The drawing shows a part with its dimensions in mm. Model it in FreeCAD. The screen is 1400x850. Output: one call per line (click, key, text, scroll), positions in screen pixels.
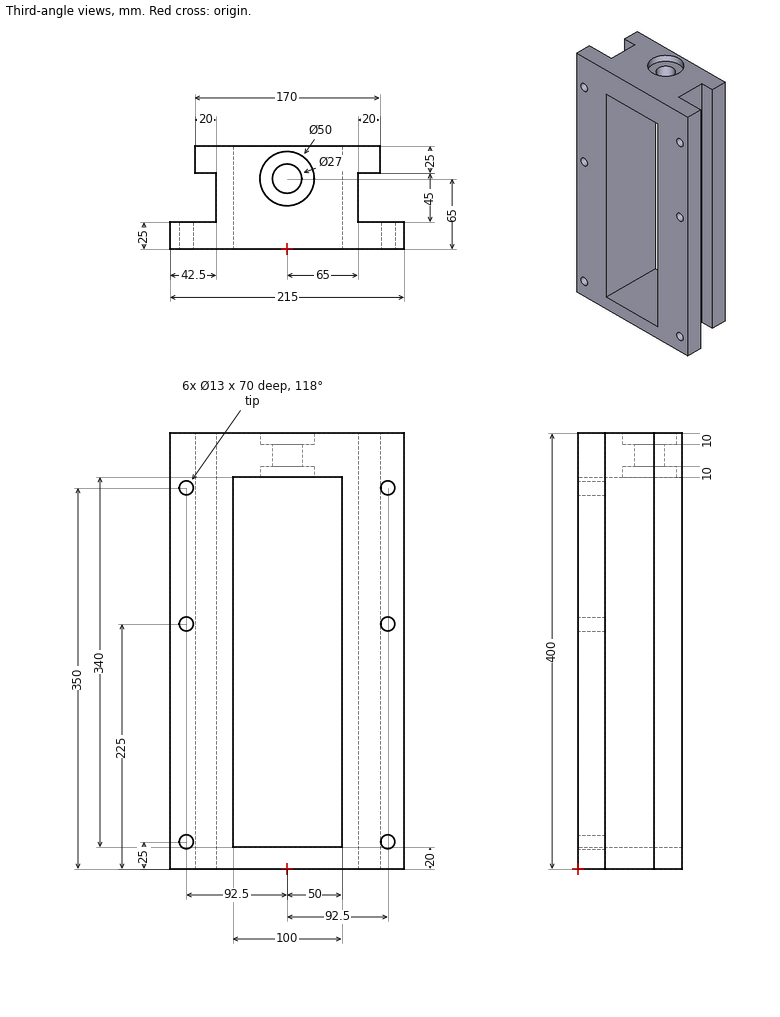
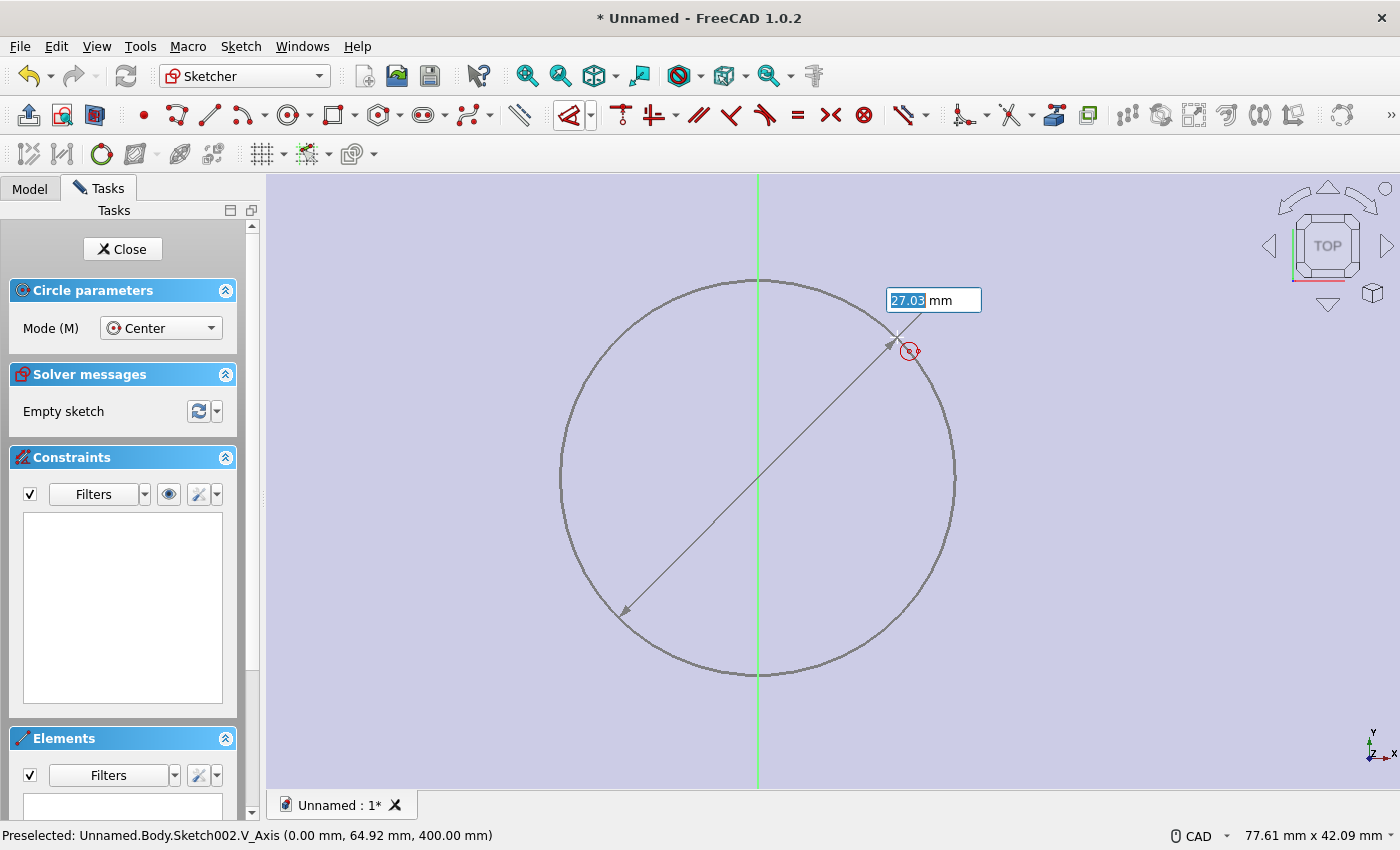
text(27)
key(Return)
key(Escape)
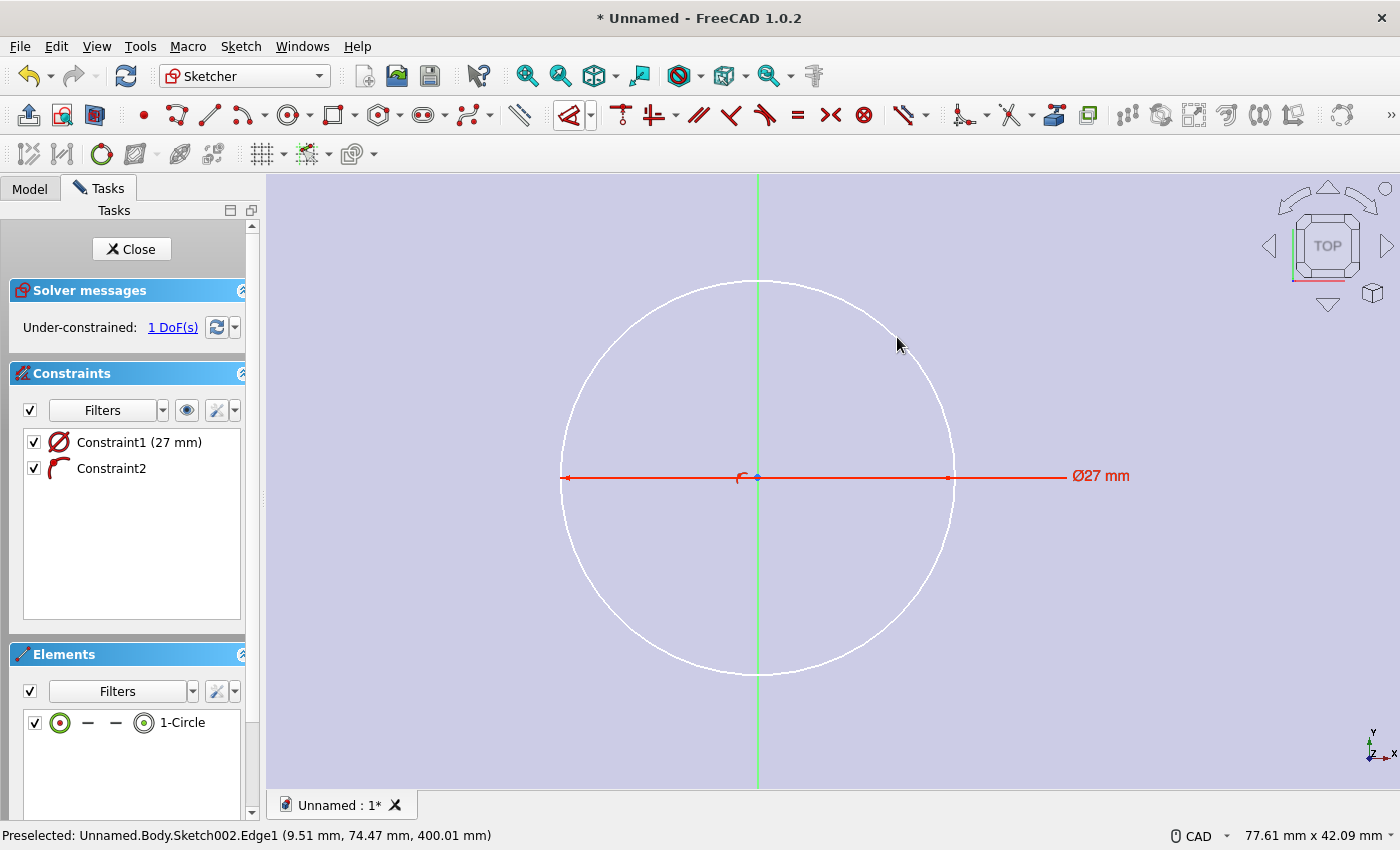
click(758, 478)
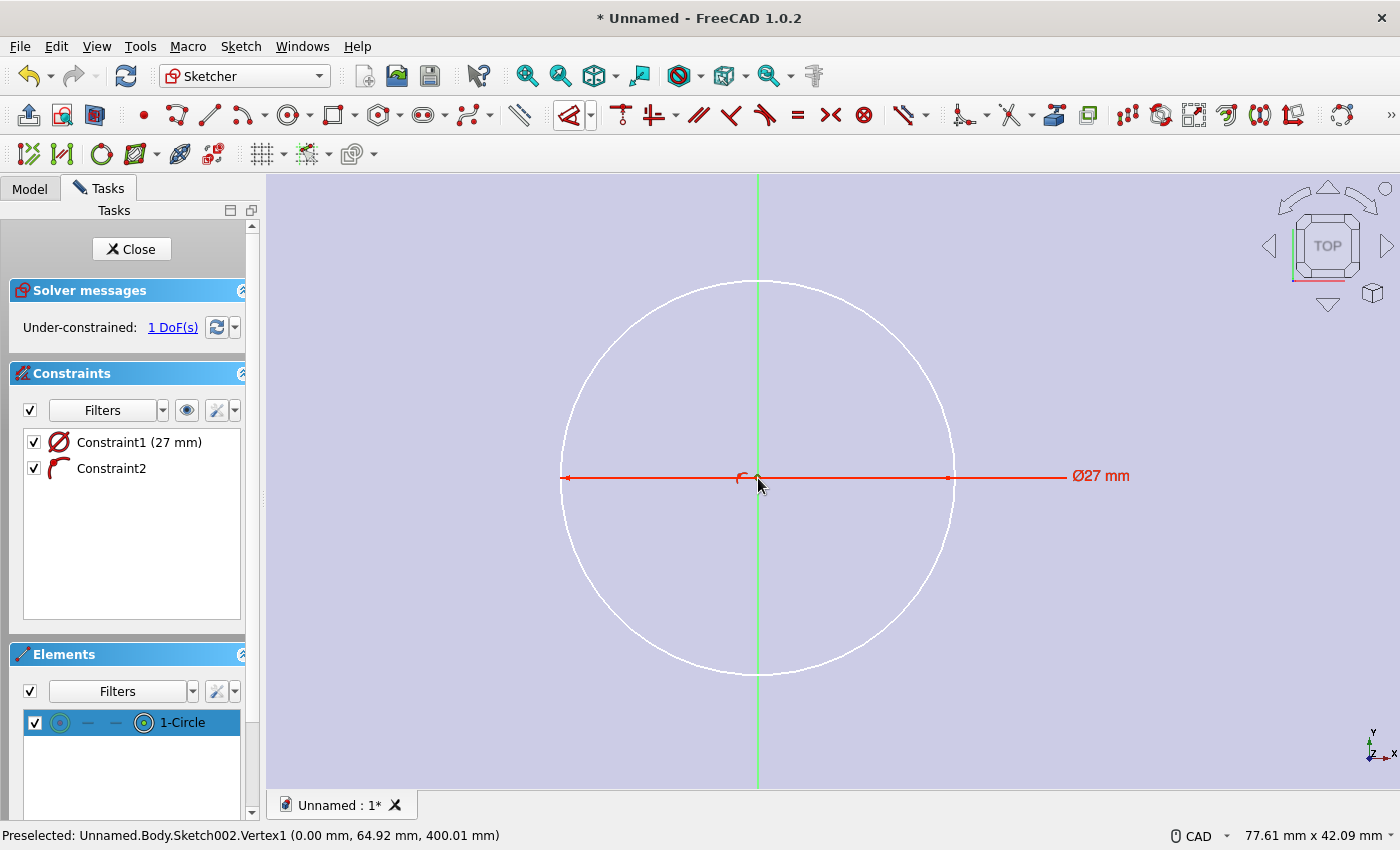
key(i)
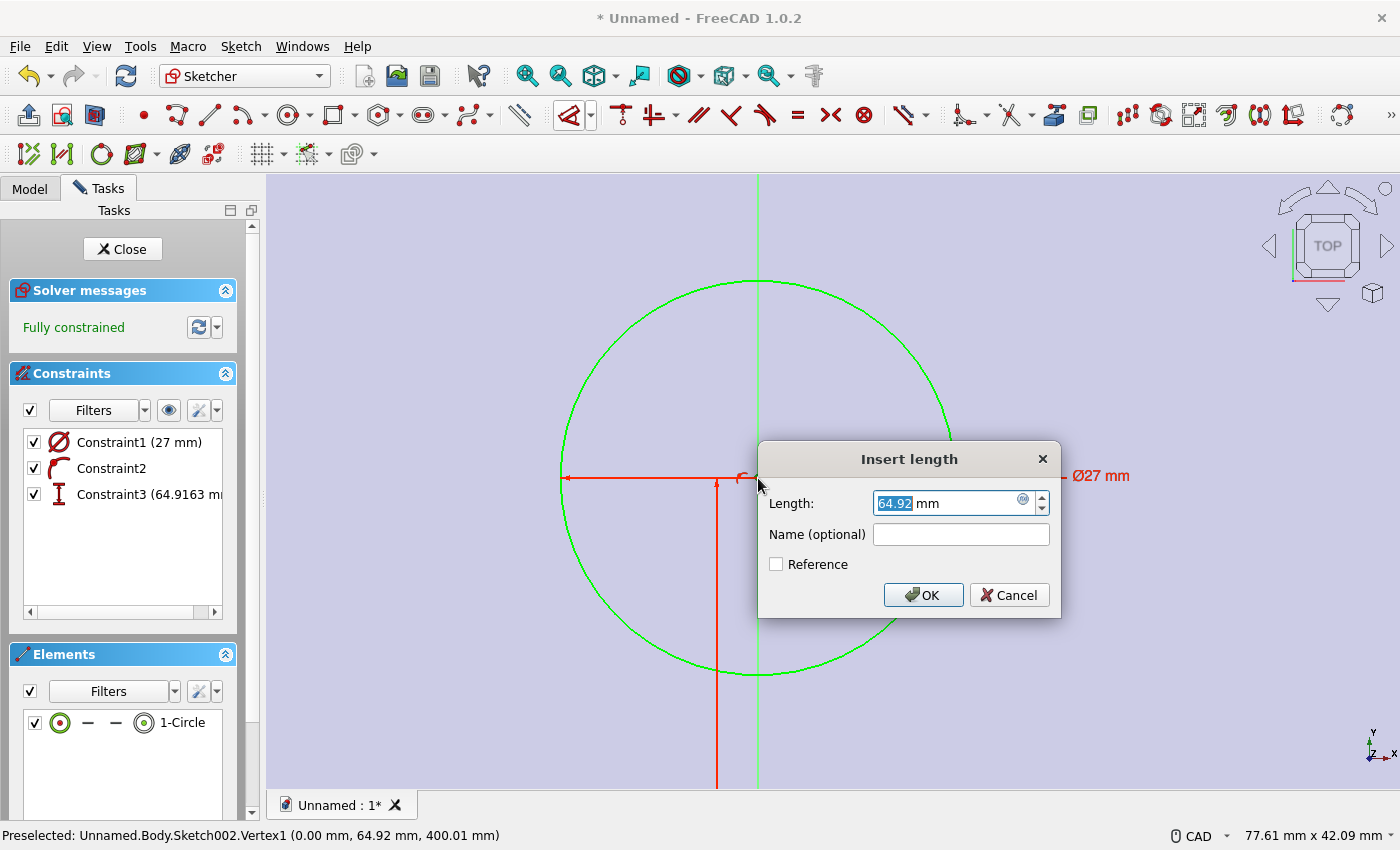
text(65)
key(Return)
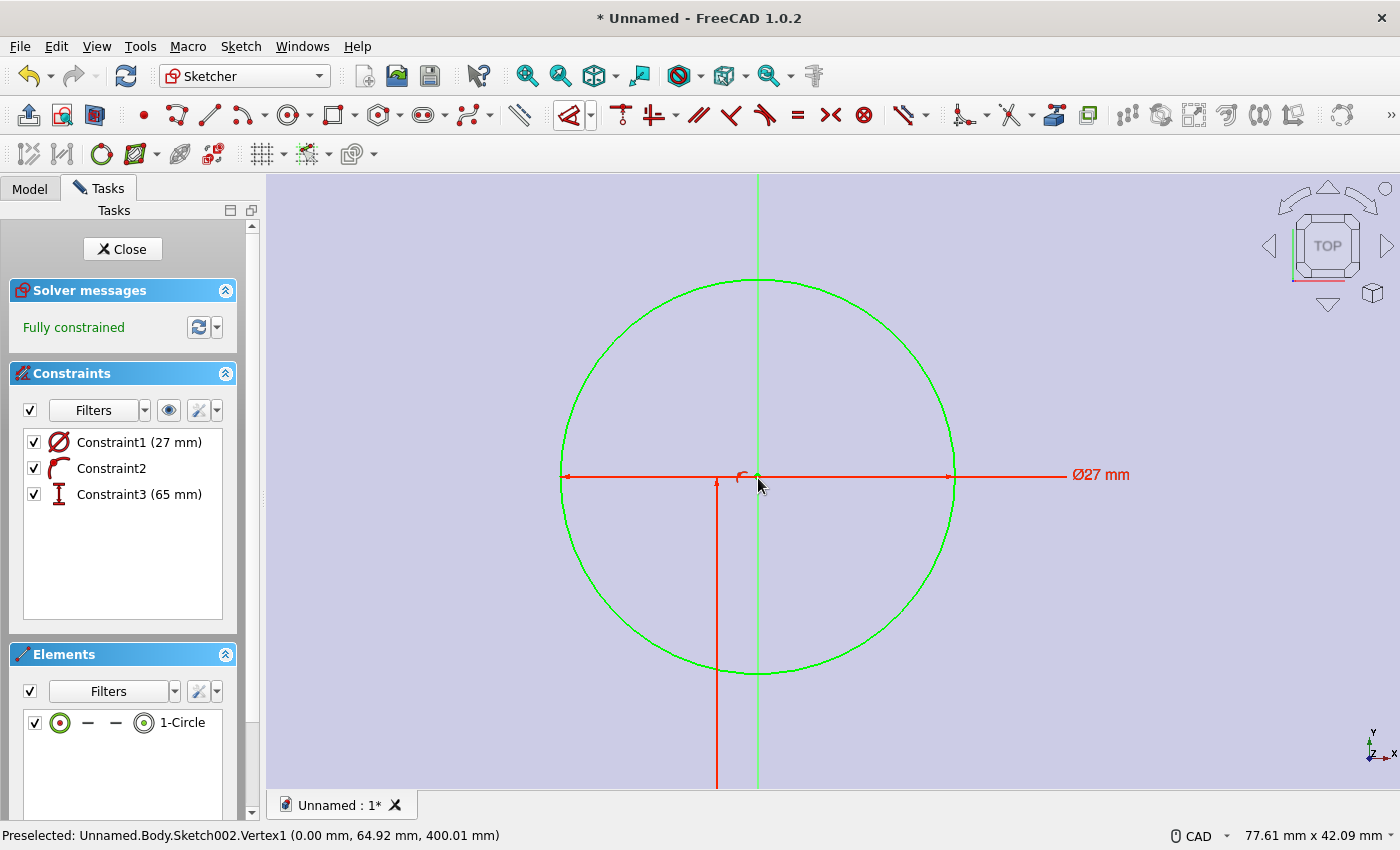
click(123, 249)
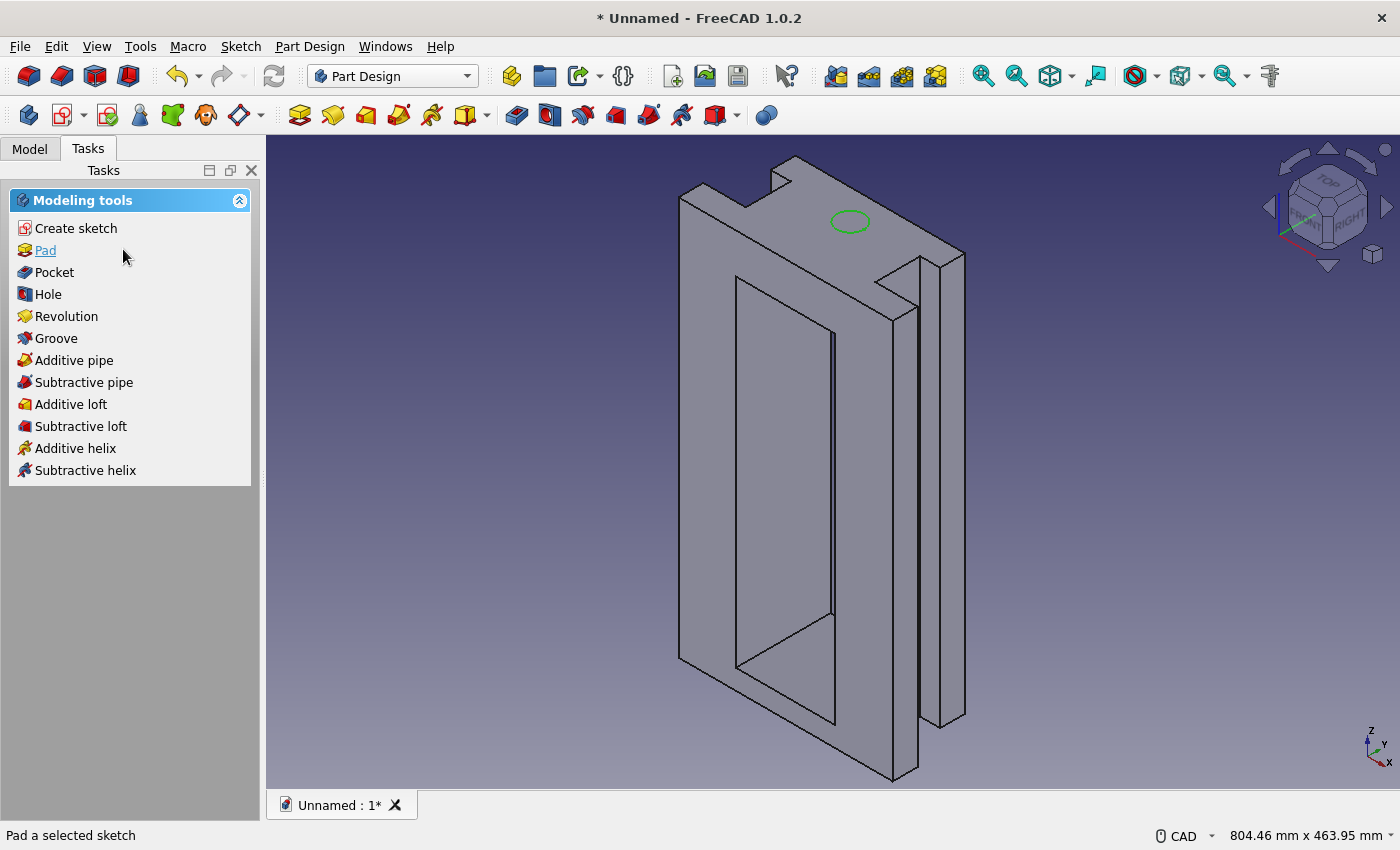
click(517, 116)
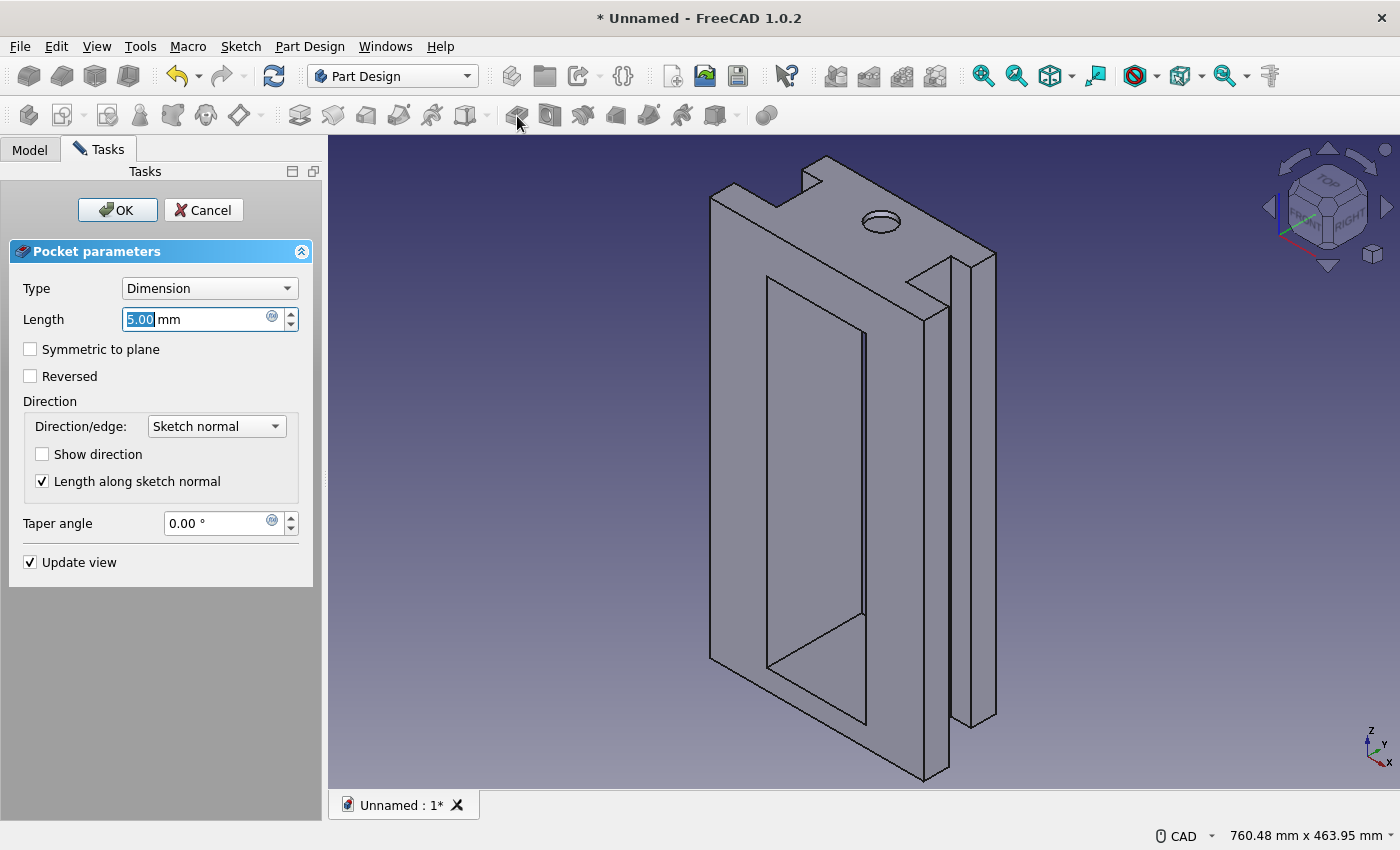
click(210, 288)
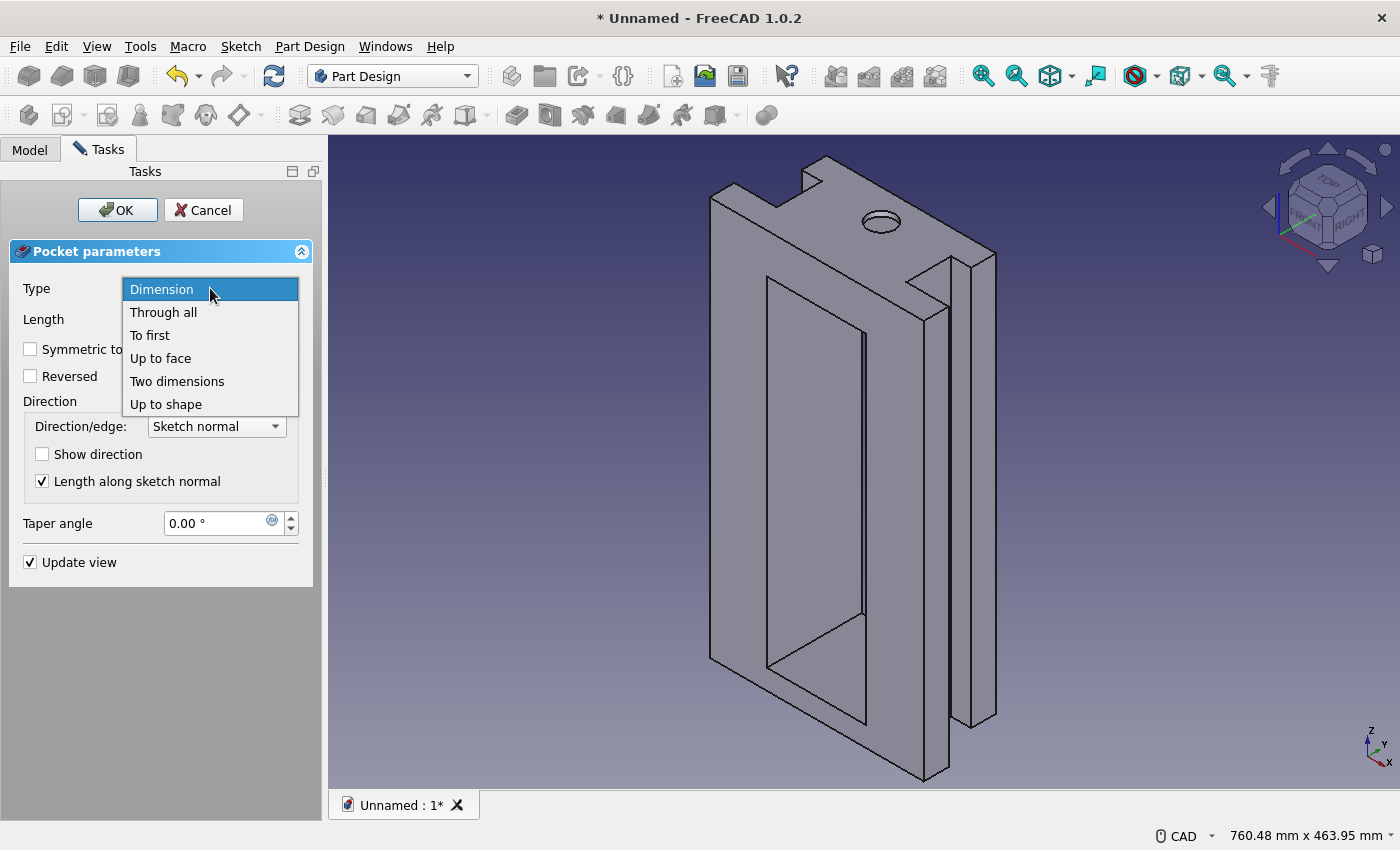
click(208, 336)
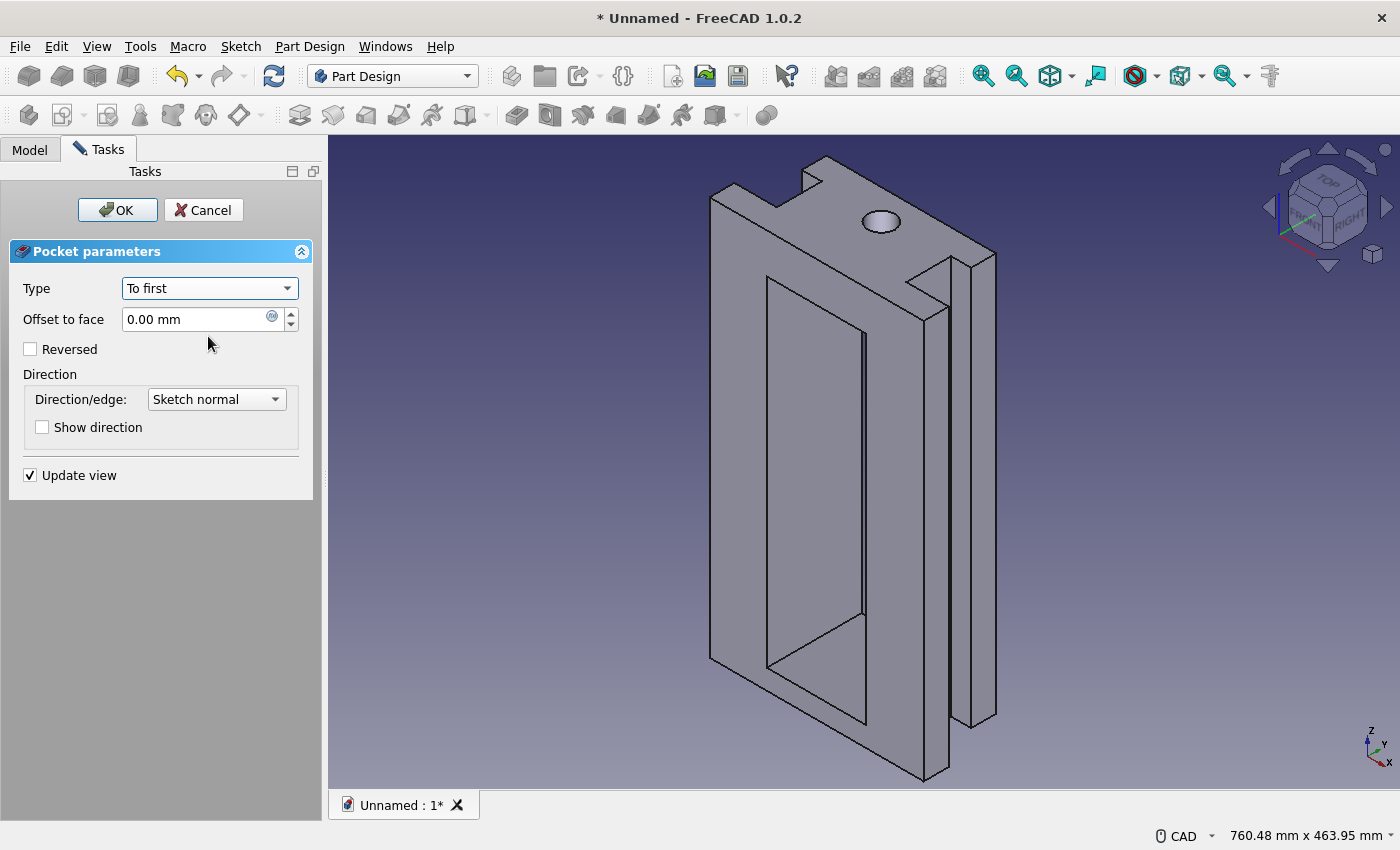
click(118, 210)